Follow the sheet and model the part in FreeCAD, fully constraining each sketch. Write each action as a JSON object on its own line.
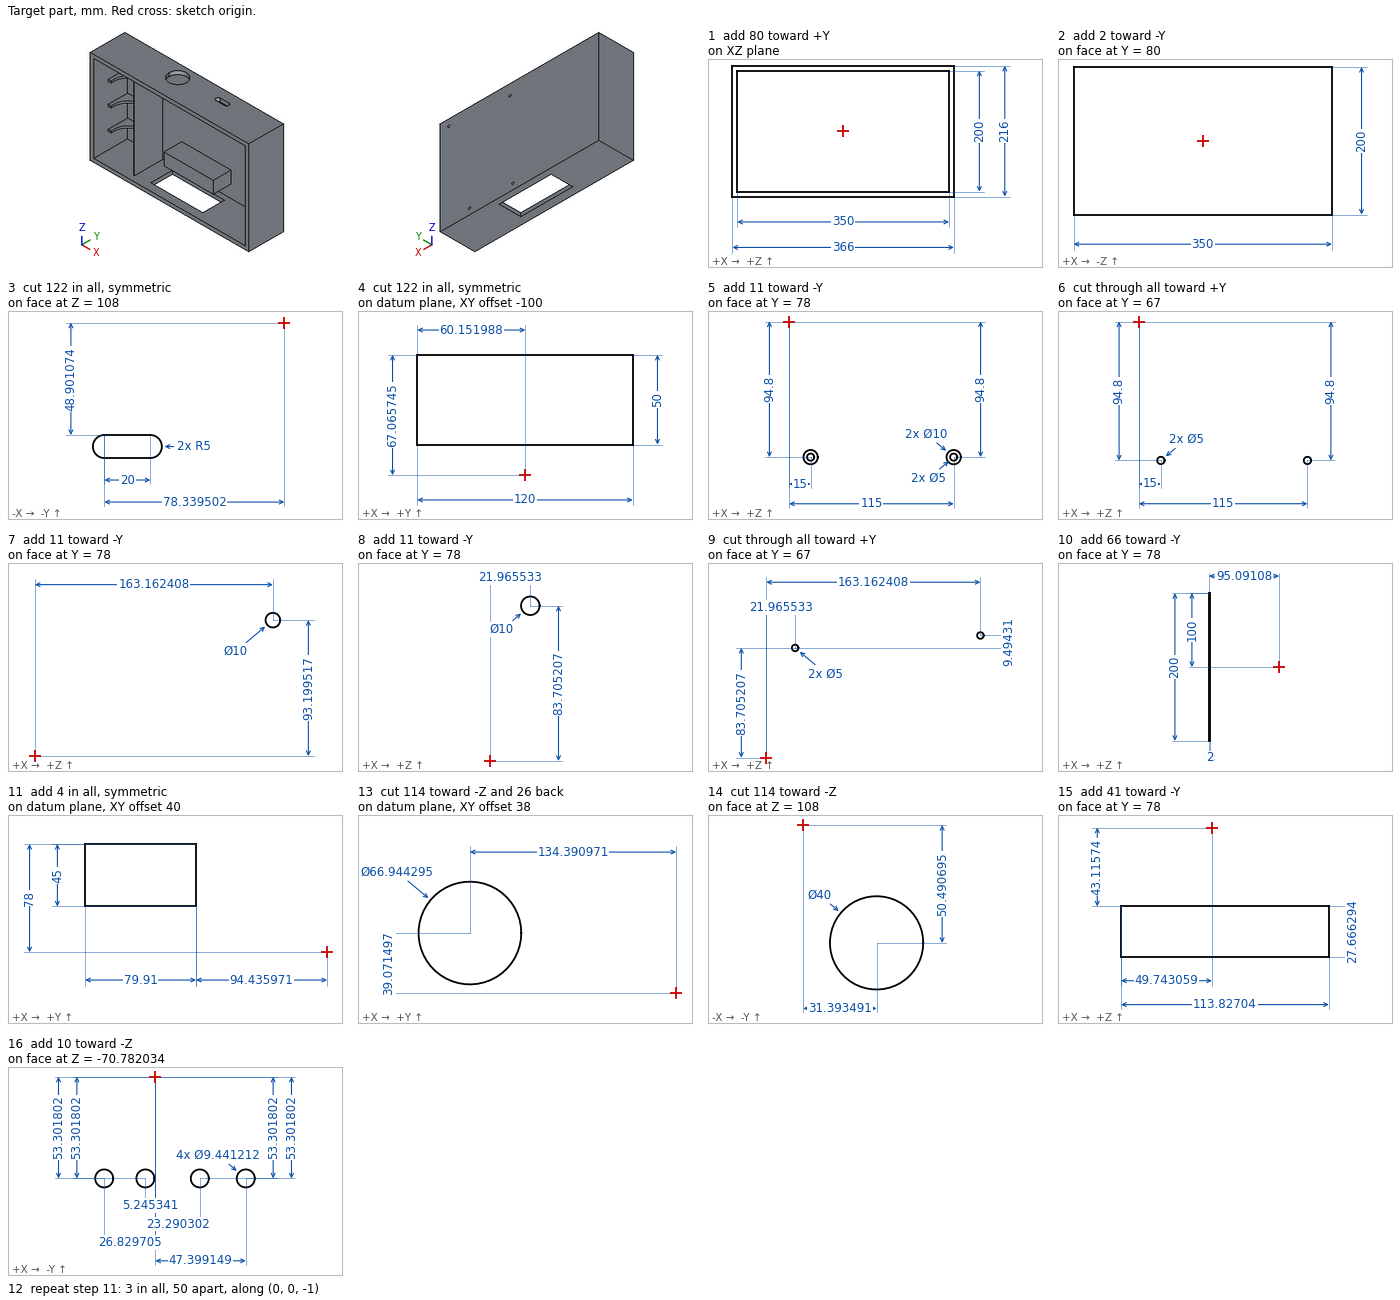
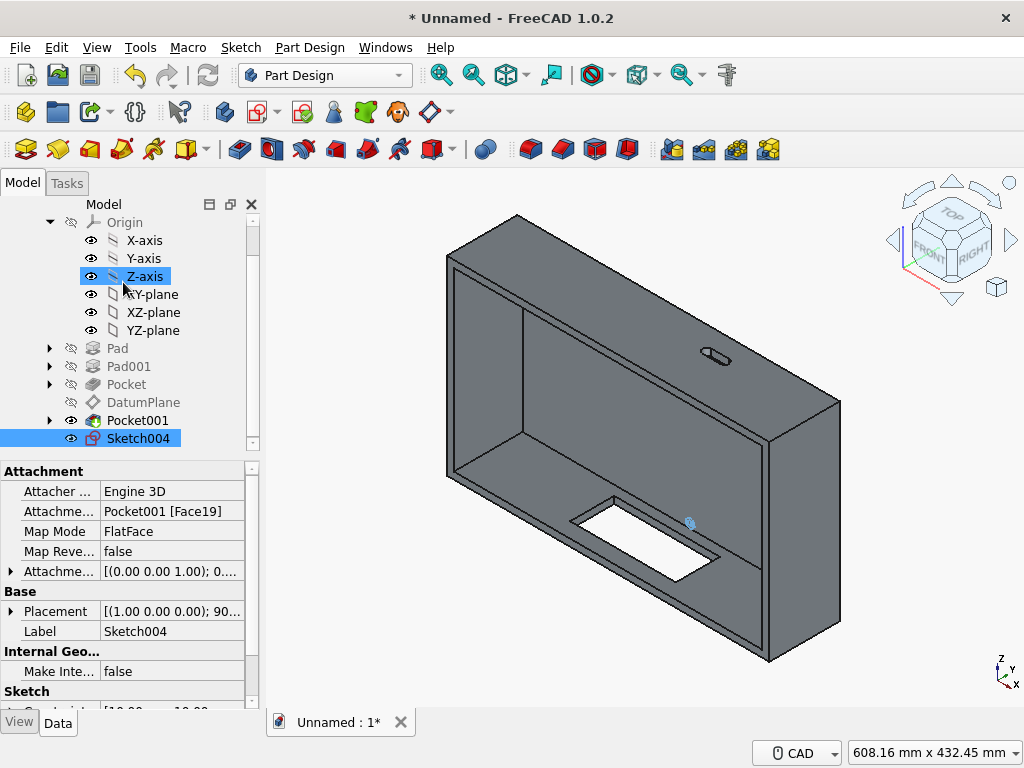
{"action": "left_click", "coordinate": [26, 150]}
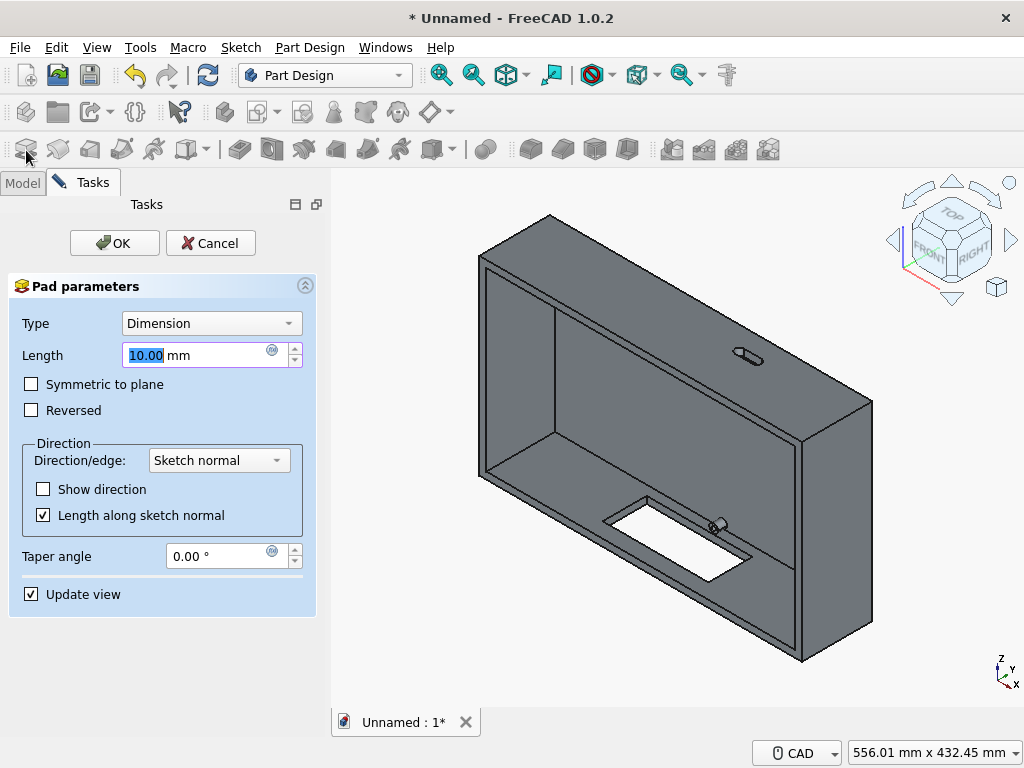
{"action": "type", "text": "11"}
{"action": "key", "text": "Tab"}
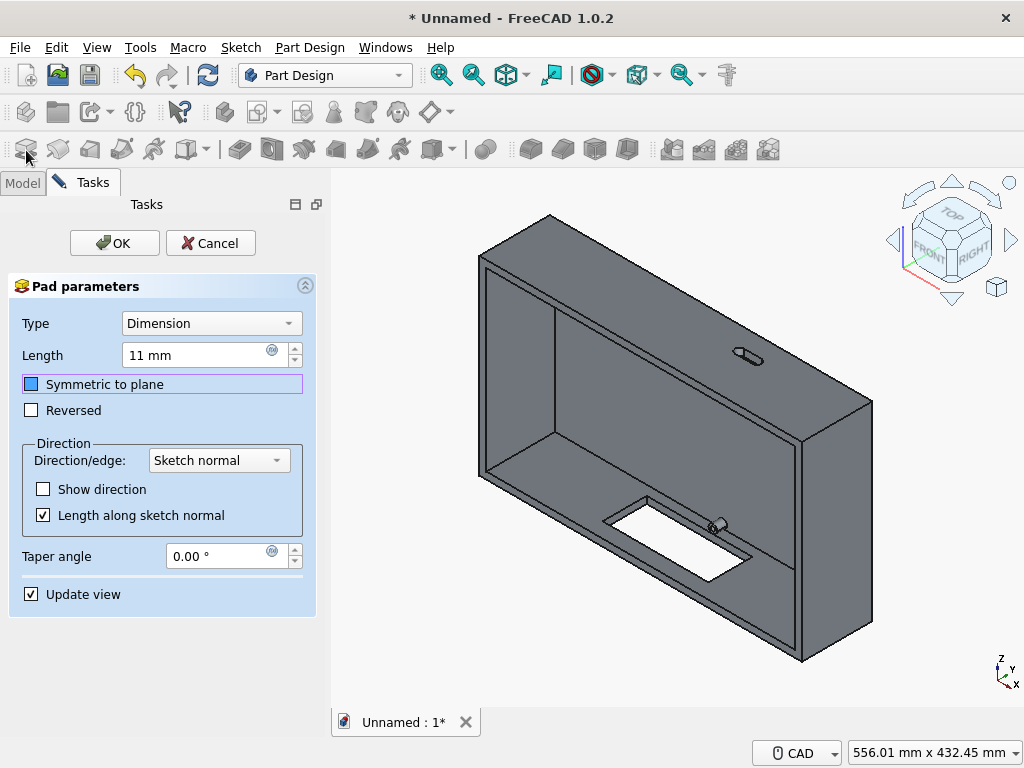
{"action": "left_click", "coordinate": [115, 243]}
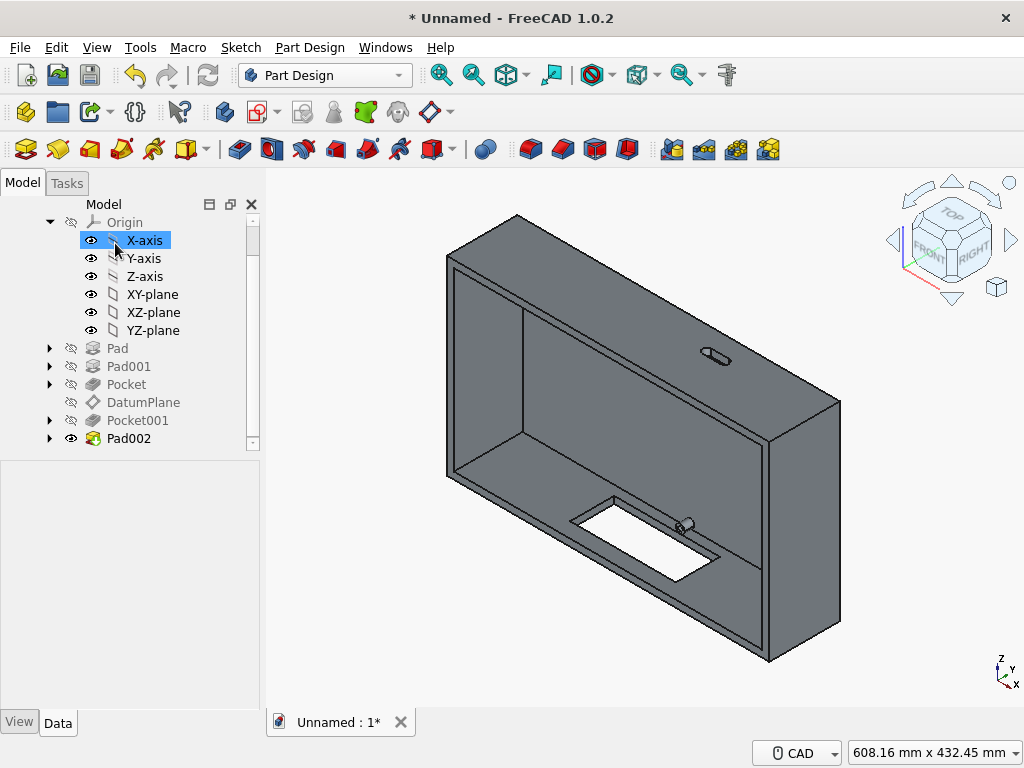
{"action": "scroll", "coordinate": [771, 577], "scroll_direction": "up", "scroll_amount": 12}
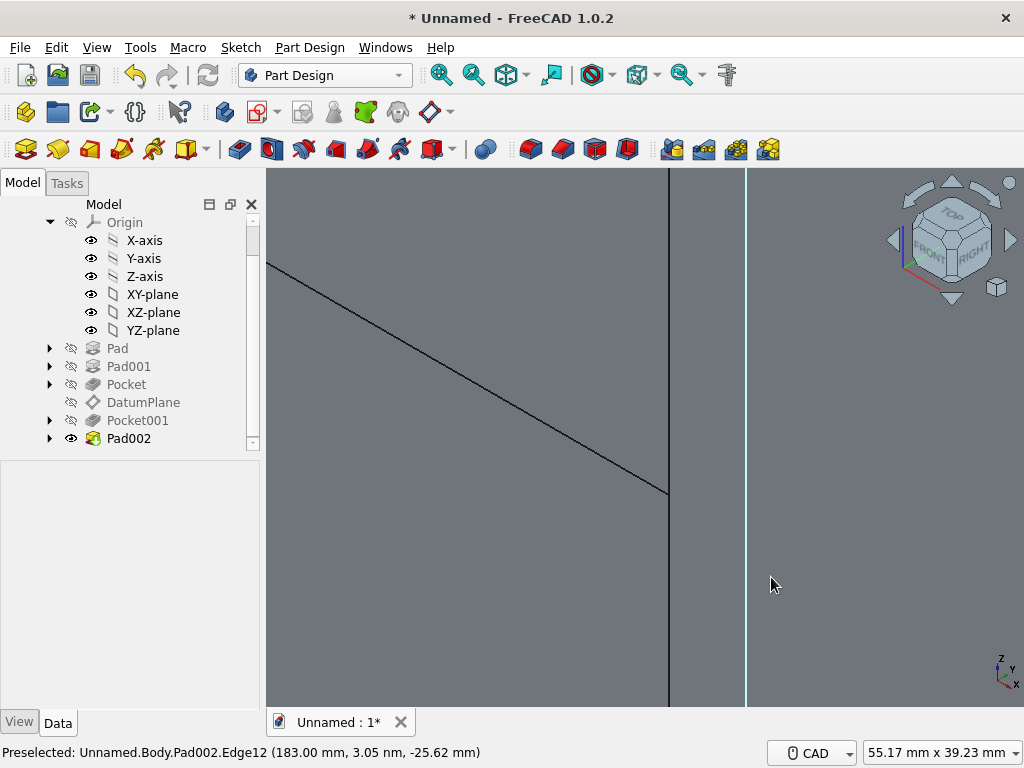
{"action": "left_click", "coordinate": [442, 76]}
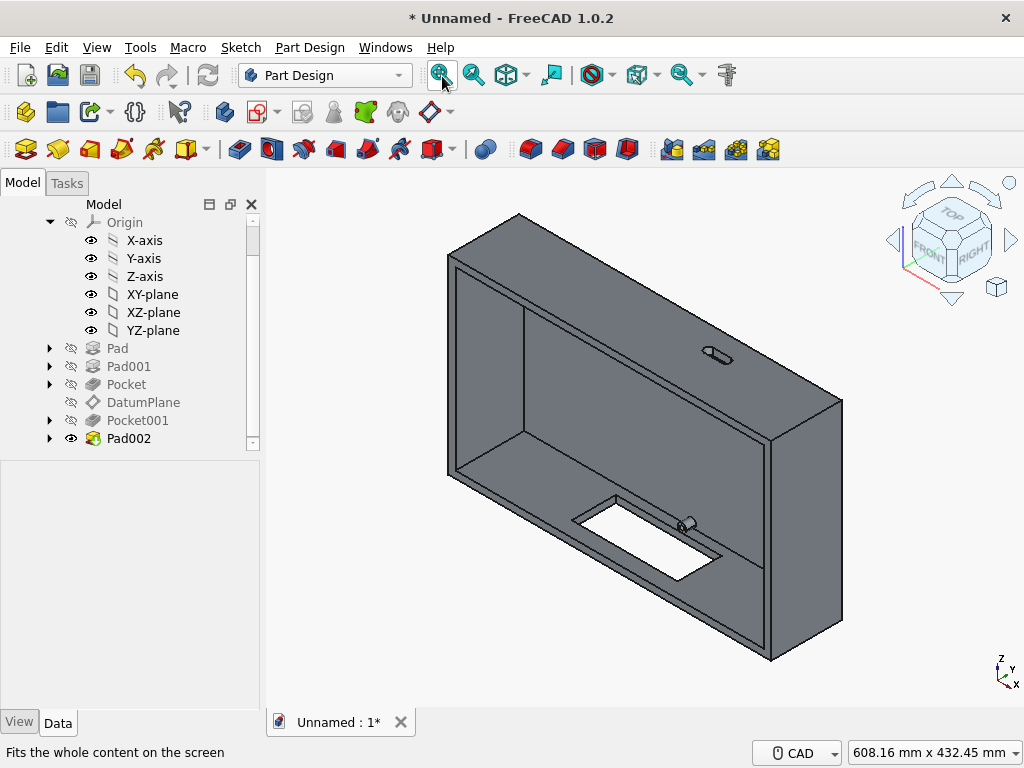
{"action": "key", "text": "1"}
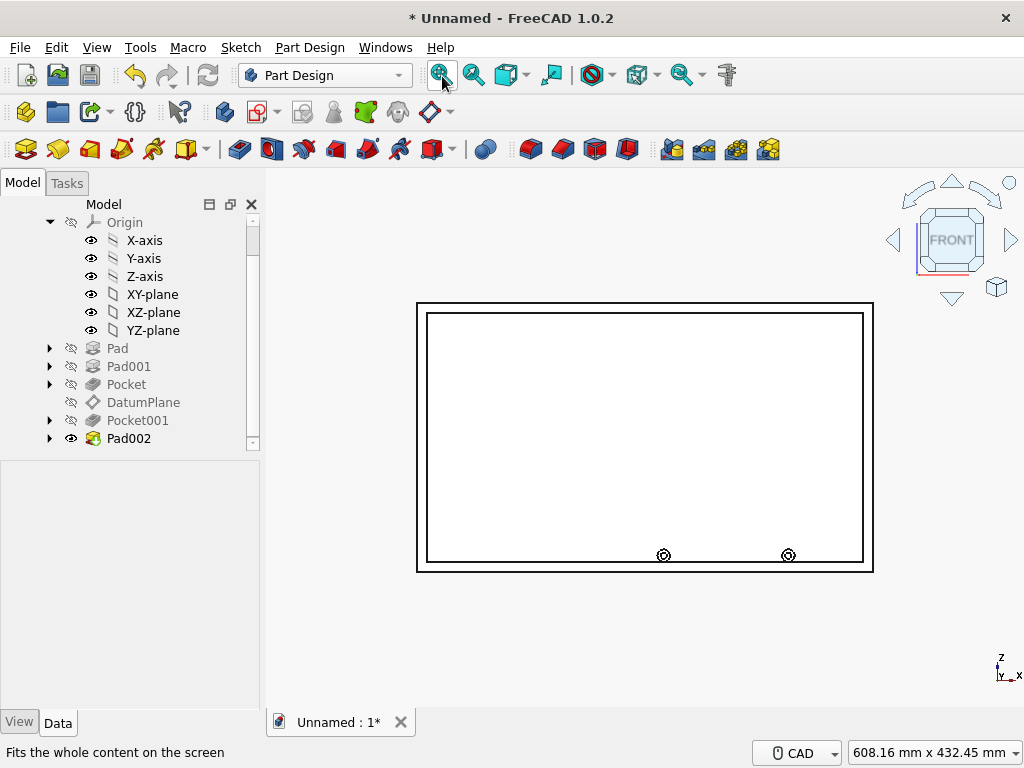
{"action": "scroll", "coordinate": [792, 551], "scroll_direction": "up", "scroll_amount": 12}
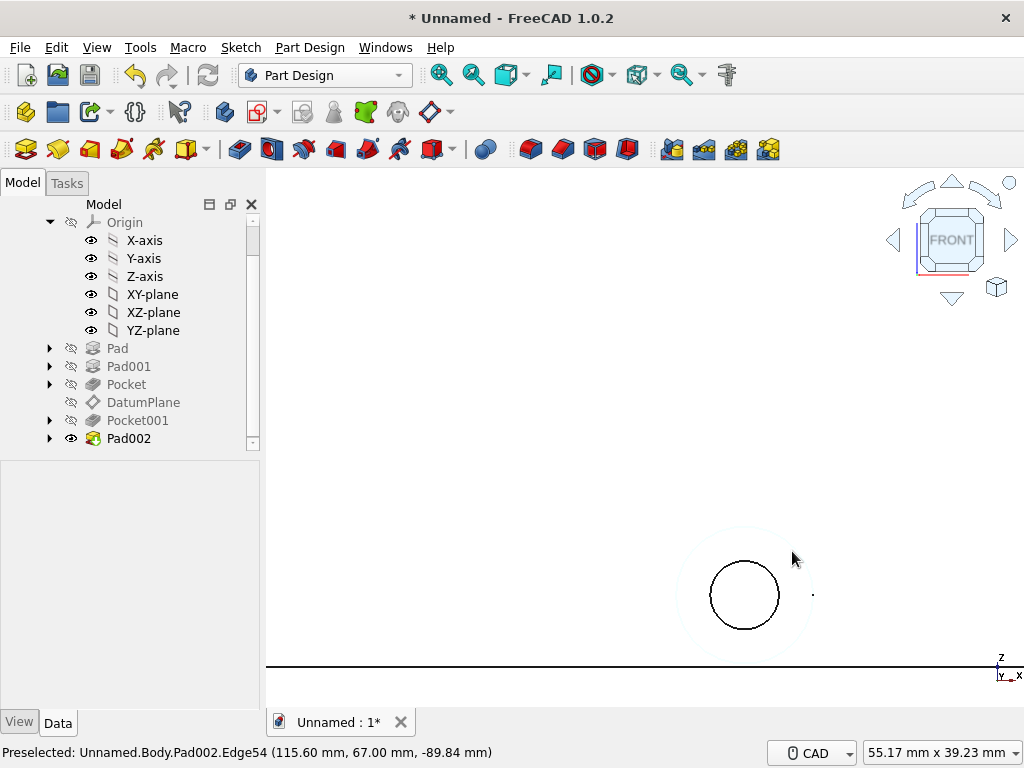
{"action": "left_click", "coordinate": [784, 555]}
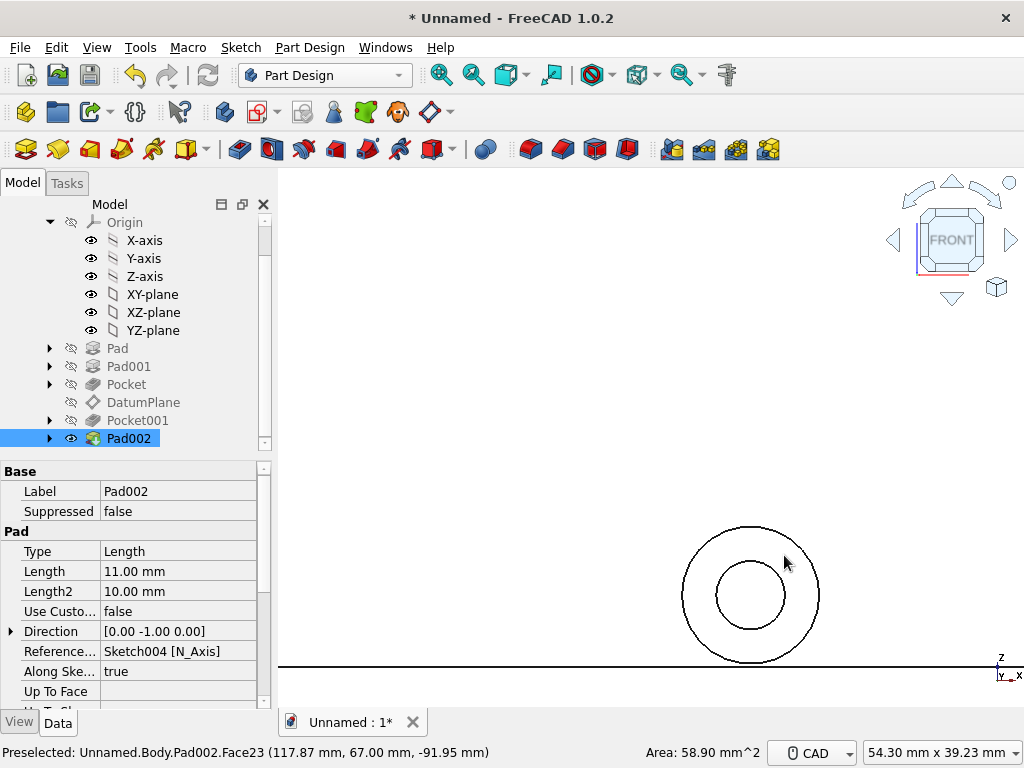
{"action": "left_click", "coordinate": [258, 112]}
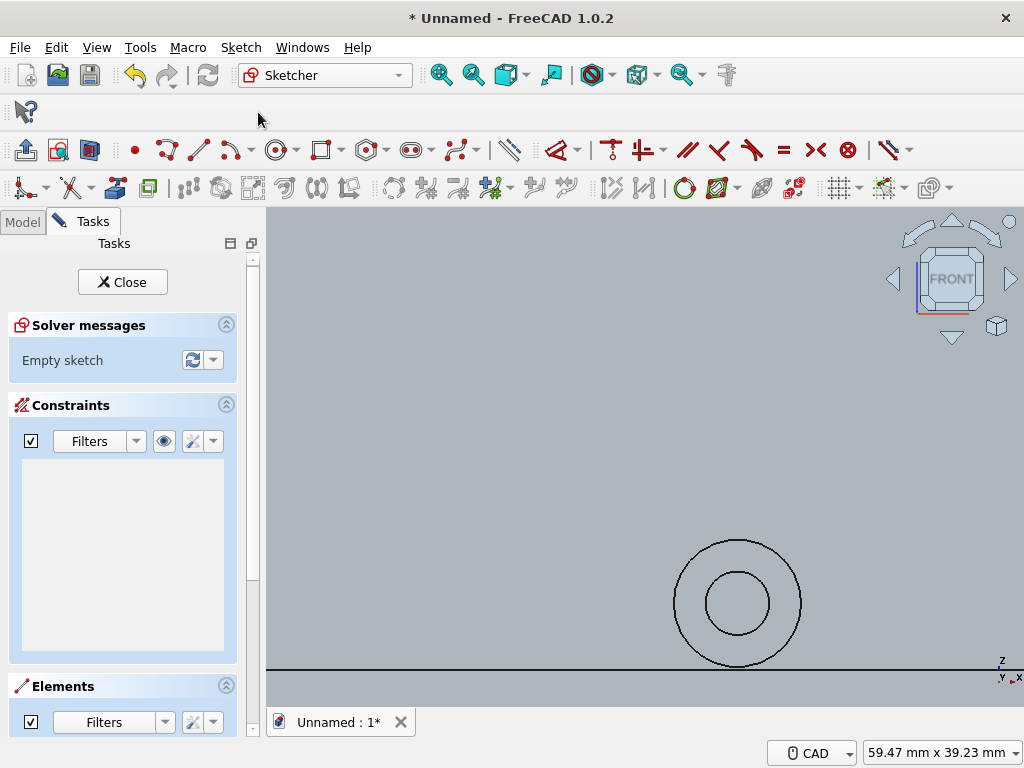
{"action": "left_click", "coordinate": [90, 150]}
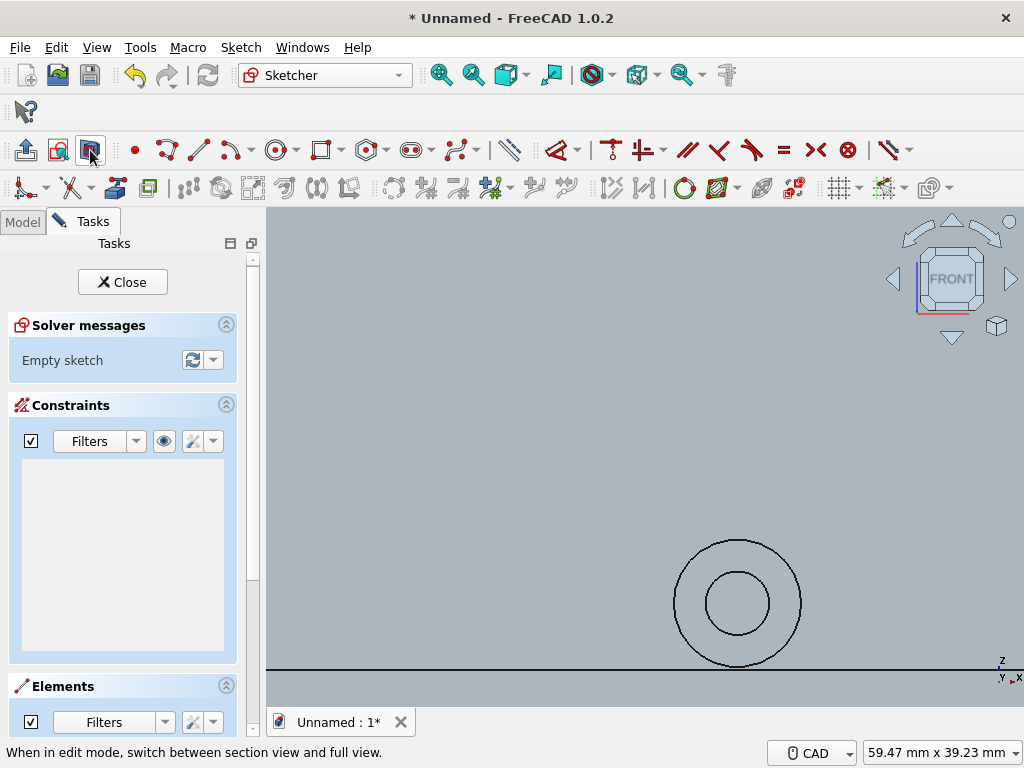
{"action": "scroll", "coordinate": [758, 602], "scroll_direction": "down", "scroll_amount": 7}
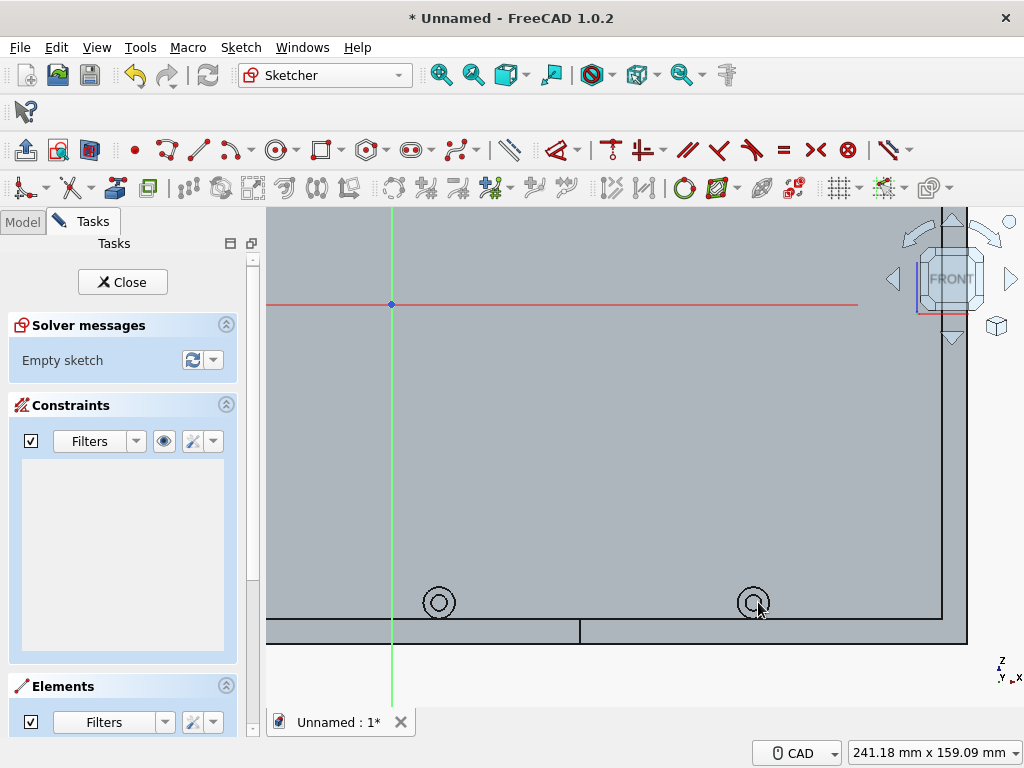
{"action": "left_click", "coordinate": [276, 150]}